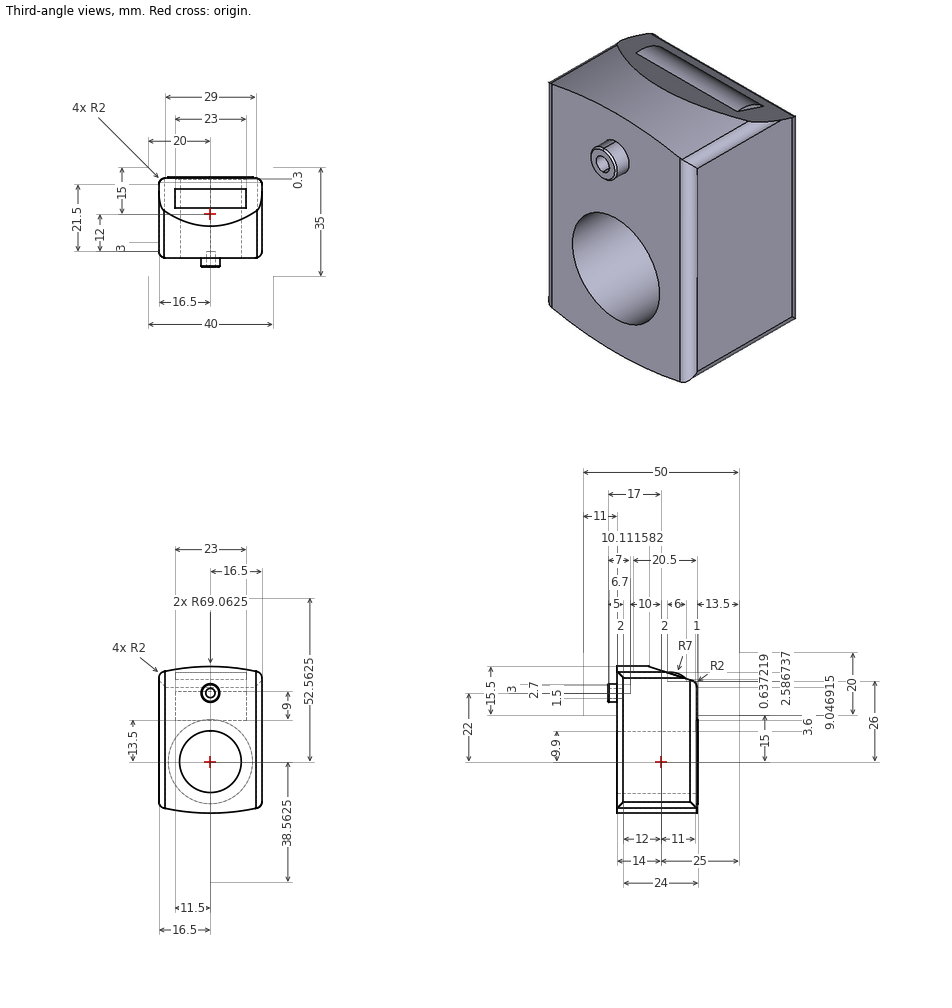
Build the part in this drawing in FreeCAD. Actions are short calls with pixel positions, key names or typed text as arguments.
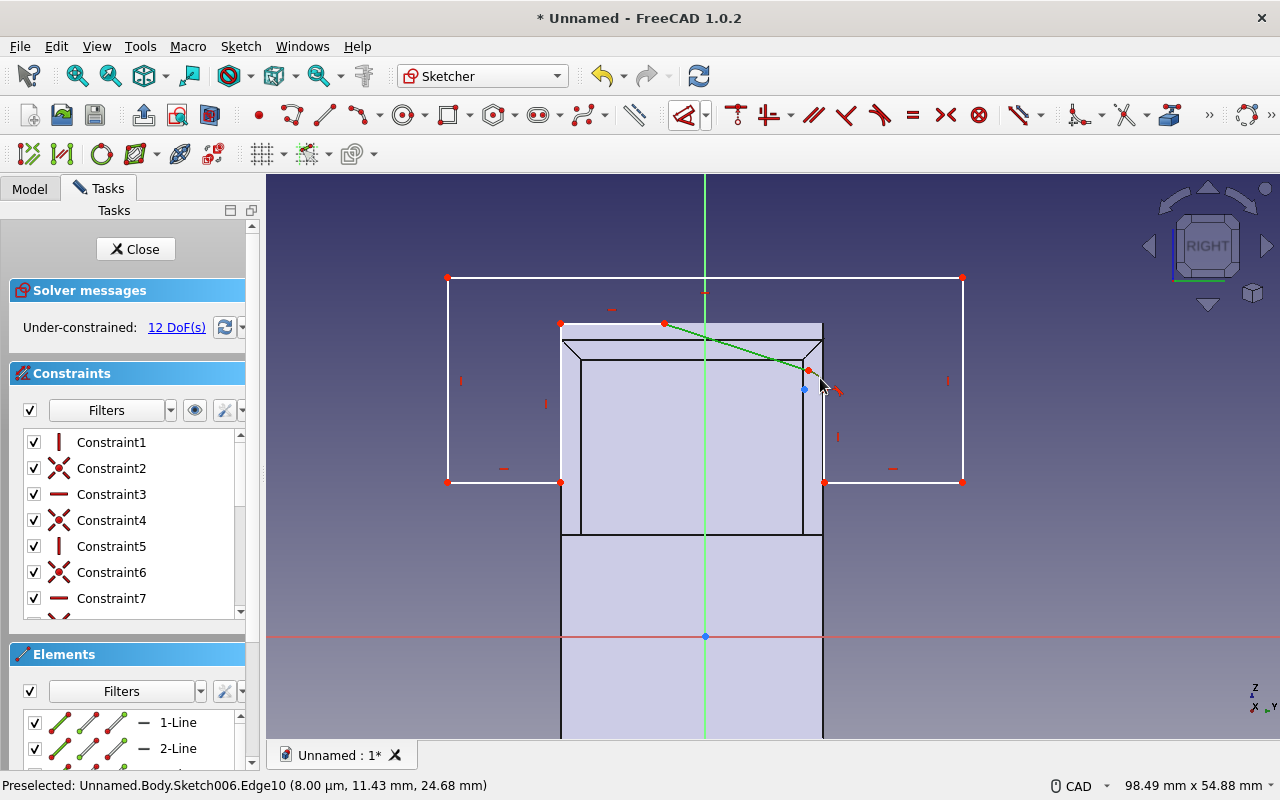
click(880, 116)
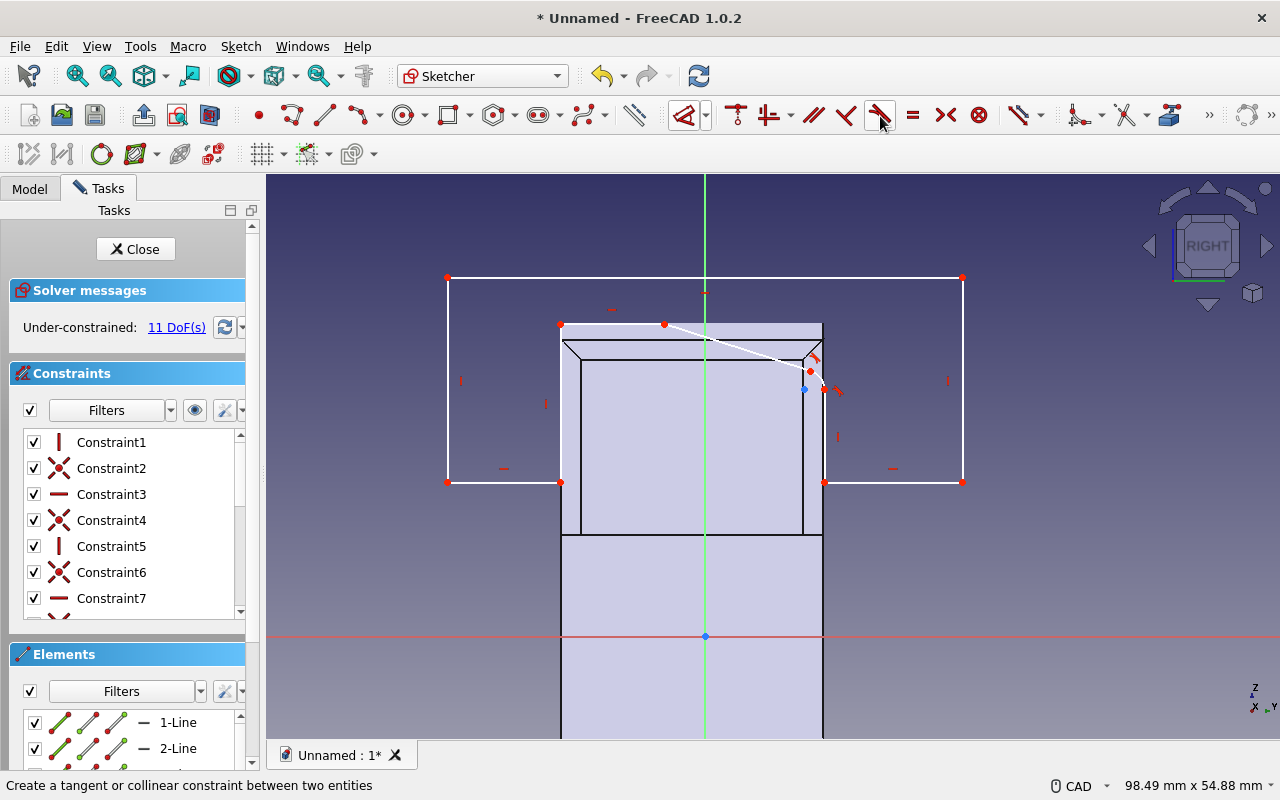
scroll(821, 378, up, 4)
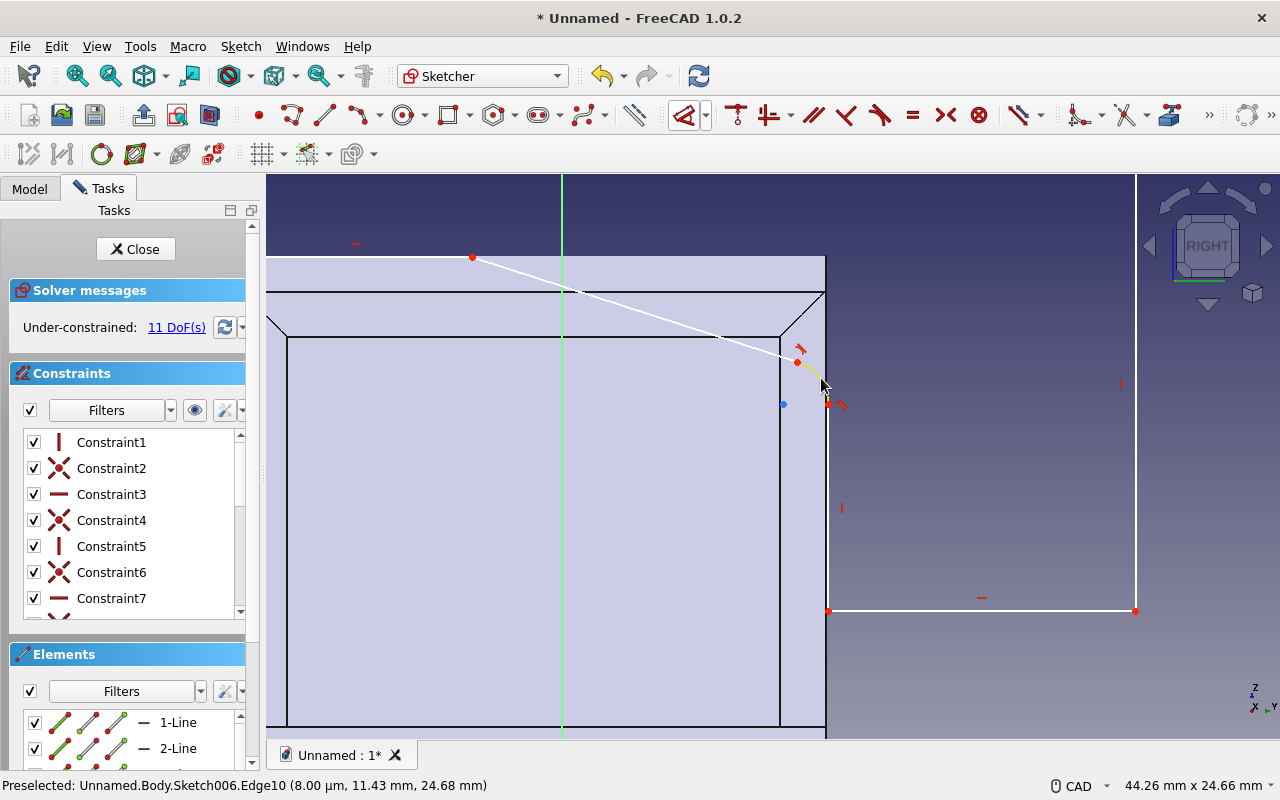
click(820, 378)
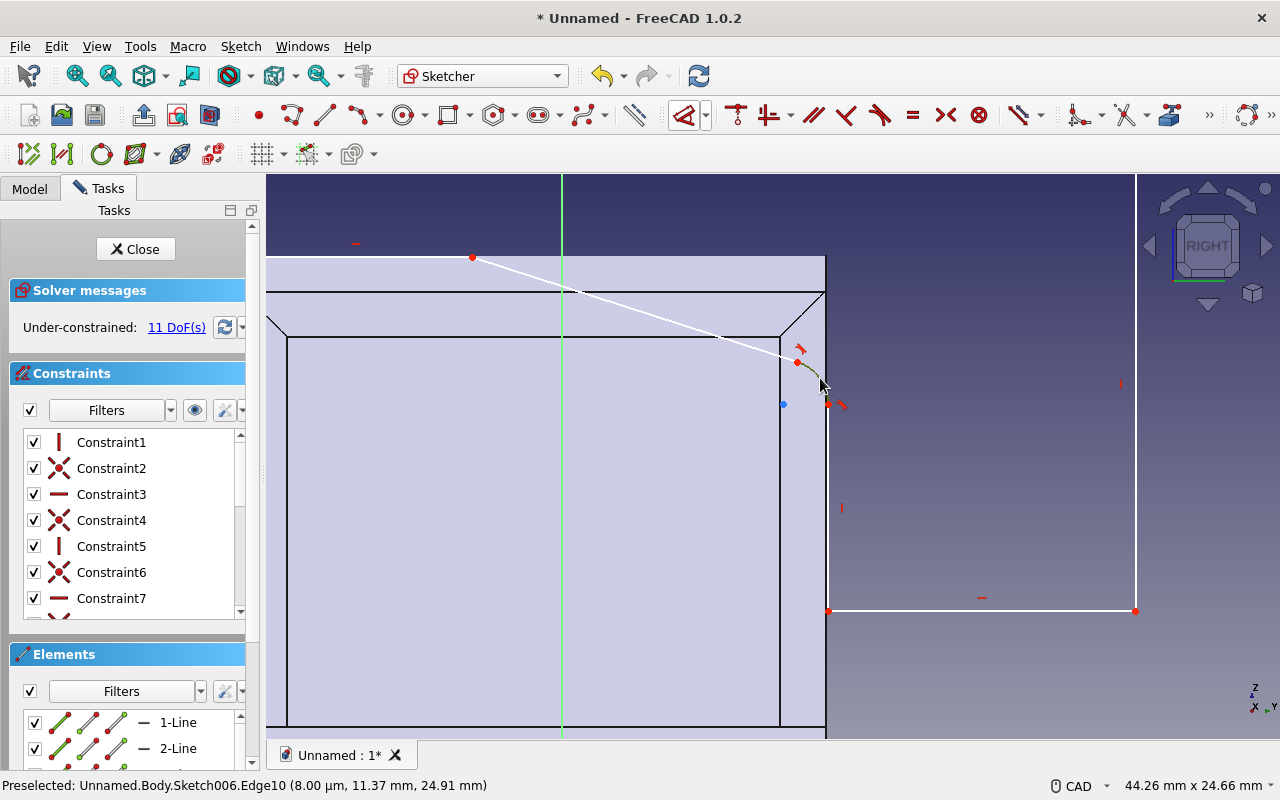
click(706, 116)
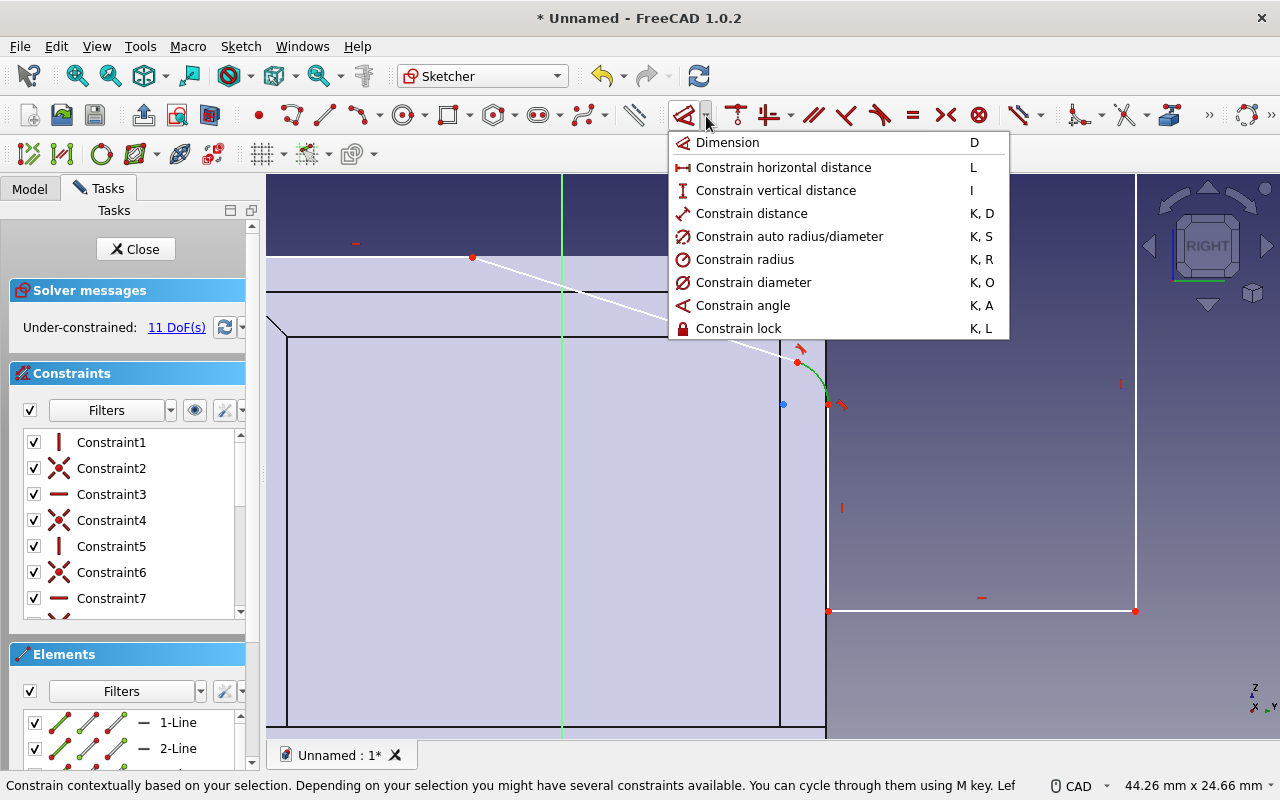
click(839, 260)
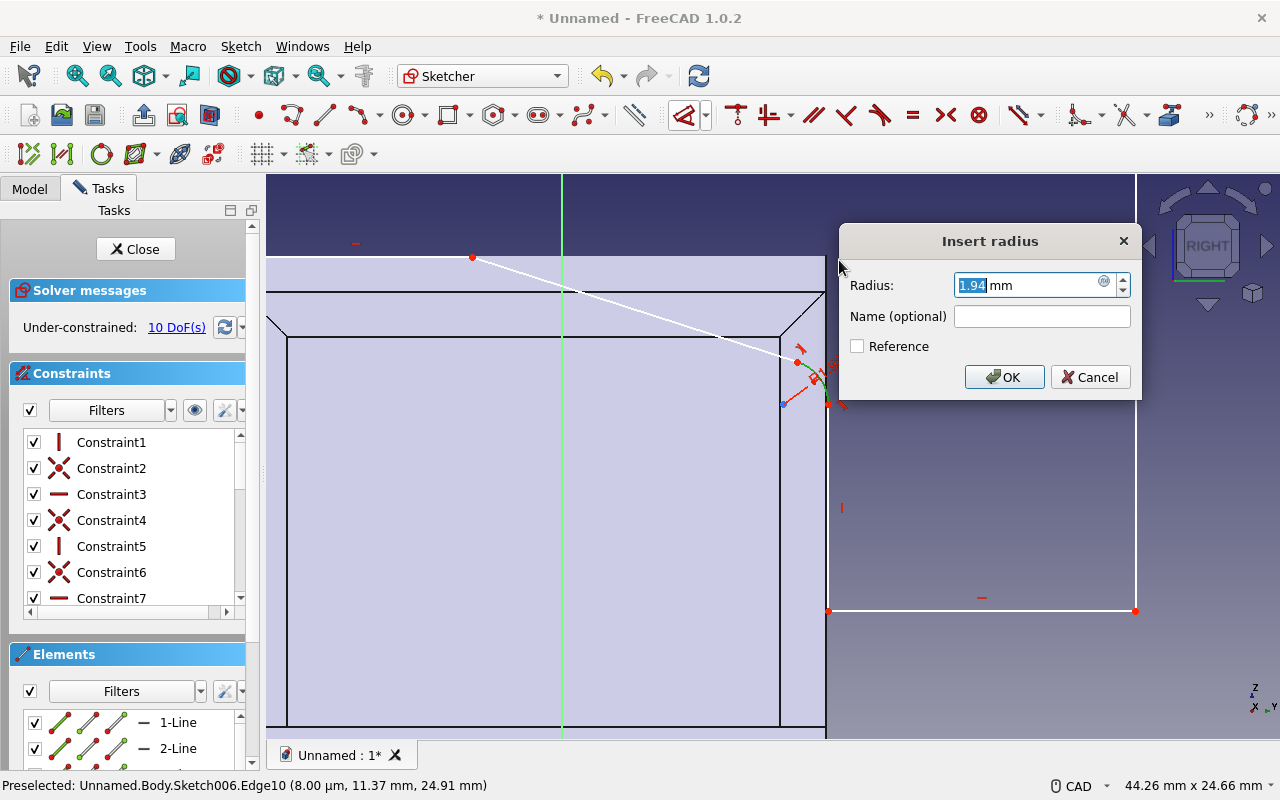
text(2)
key(Return)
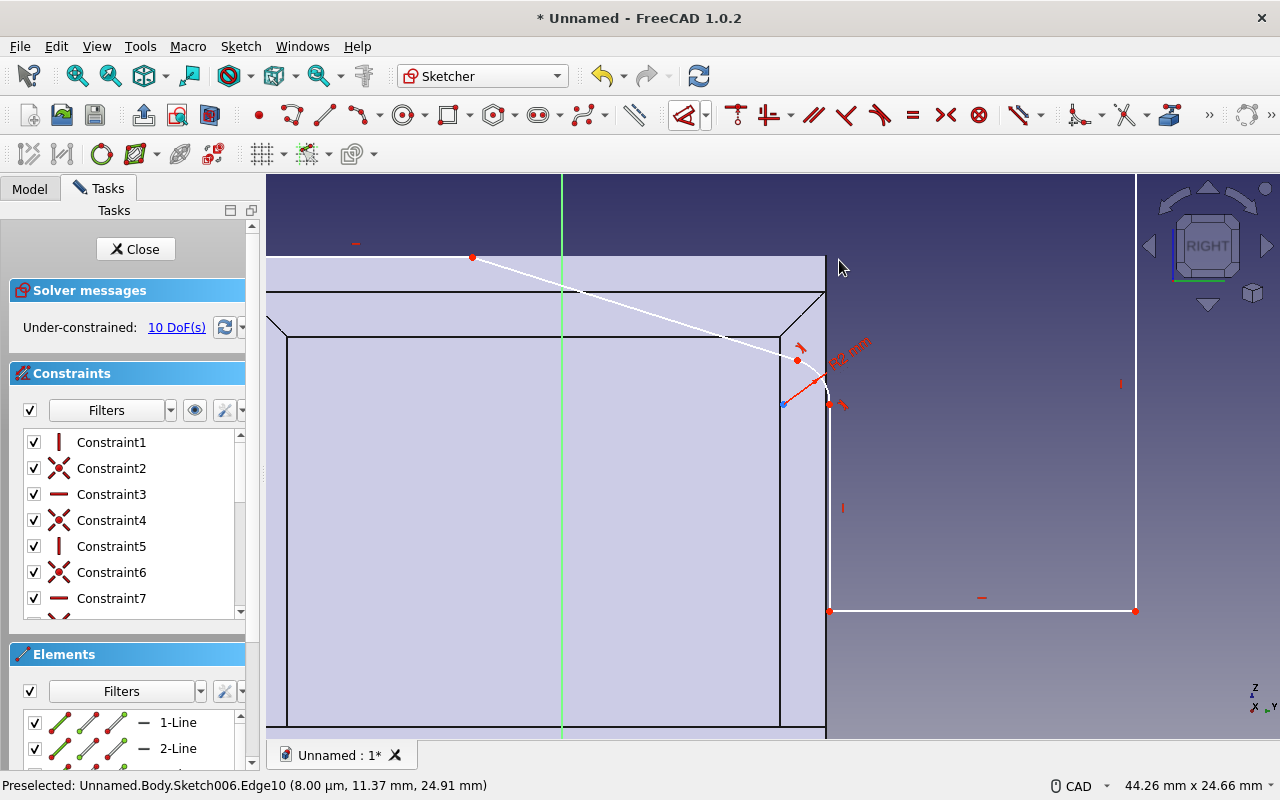
scroll(821, 378, down, 4)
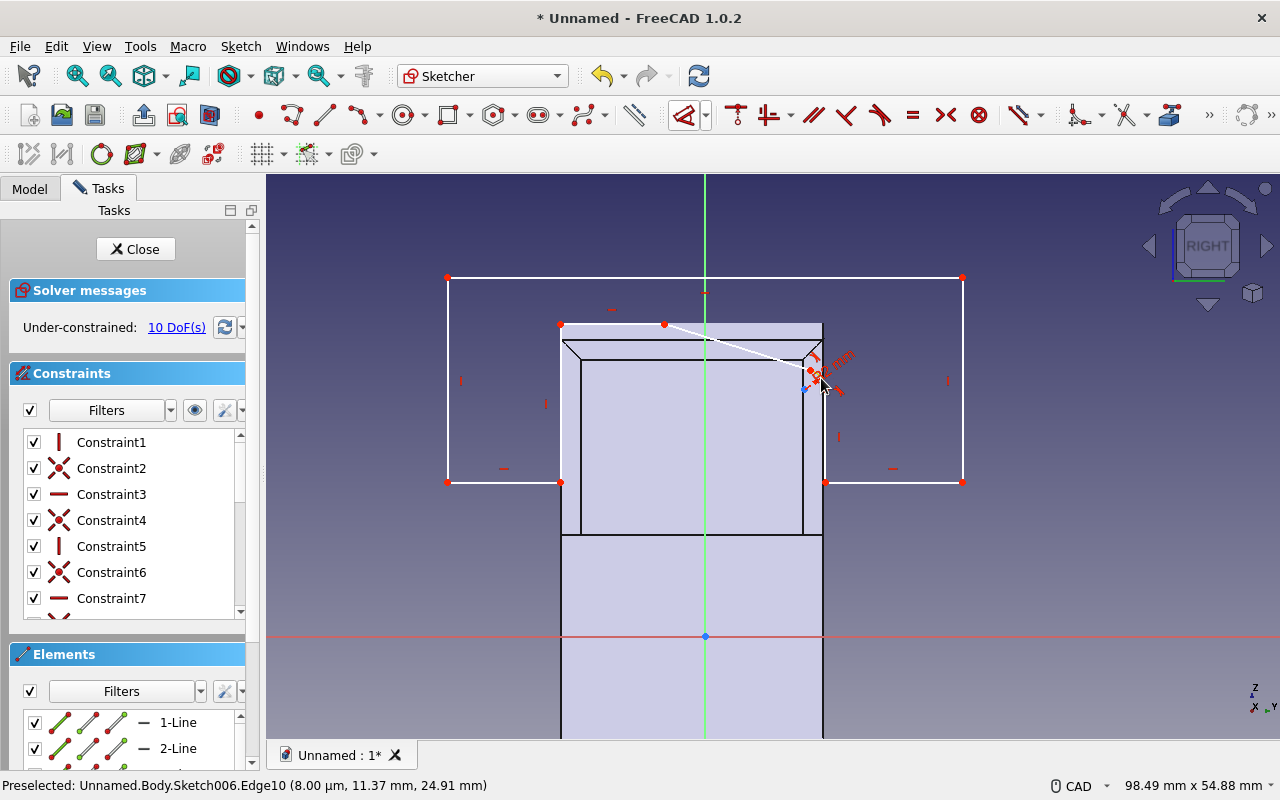
click(963, 422)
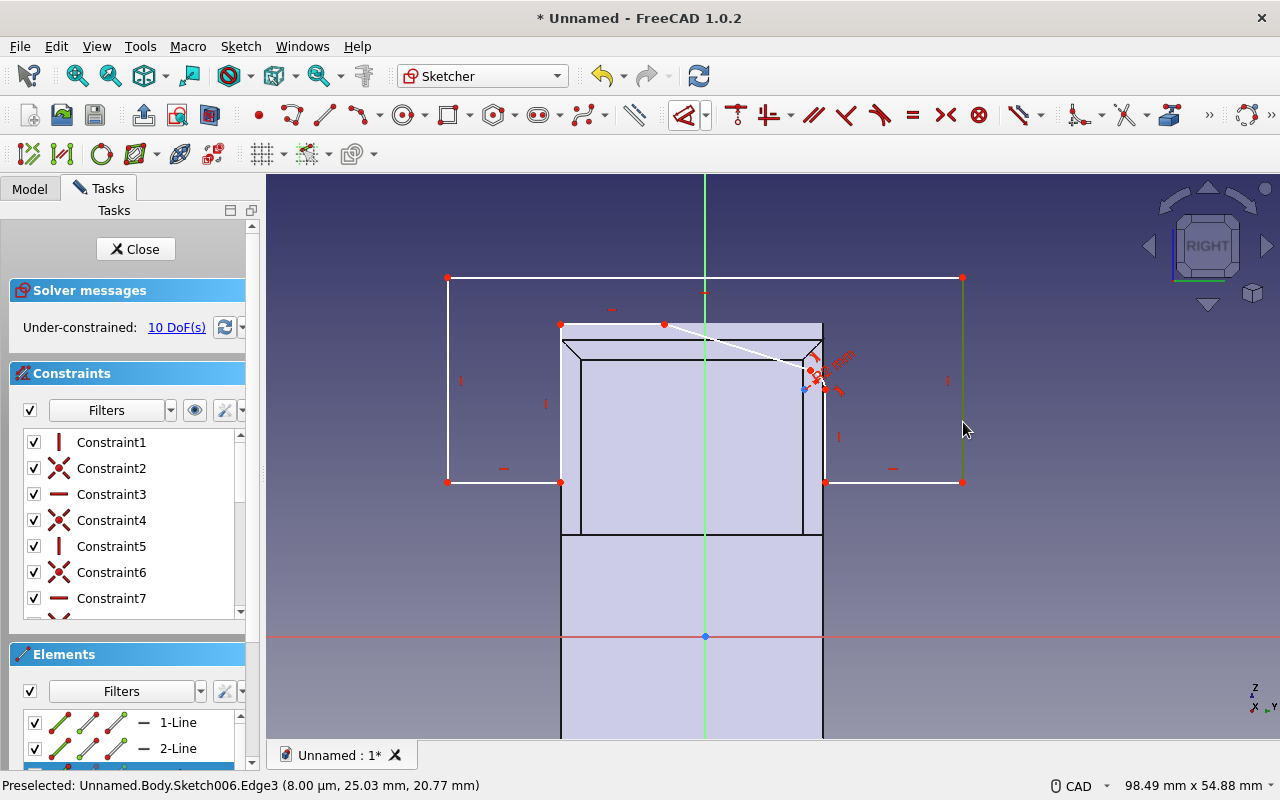
key(i)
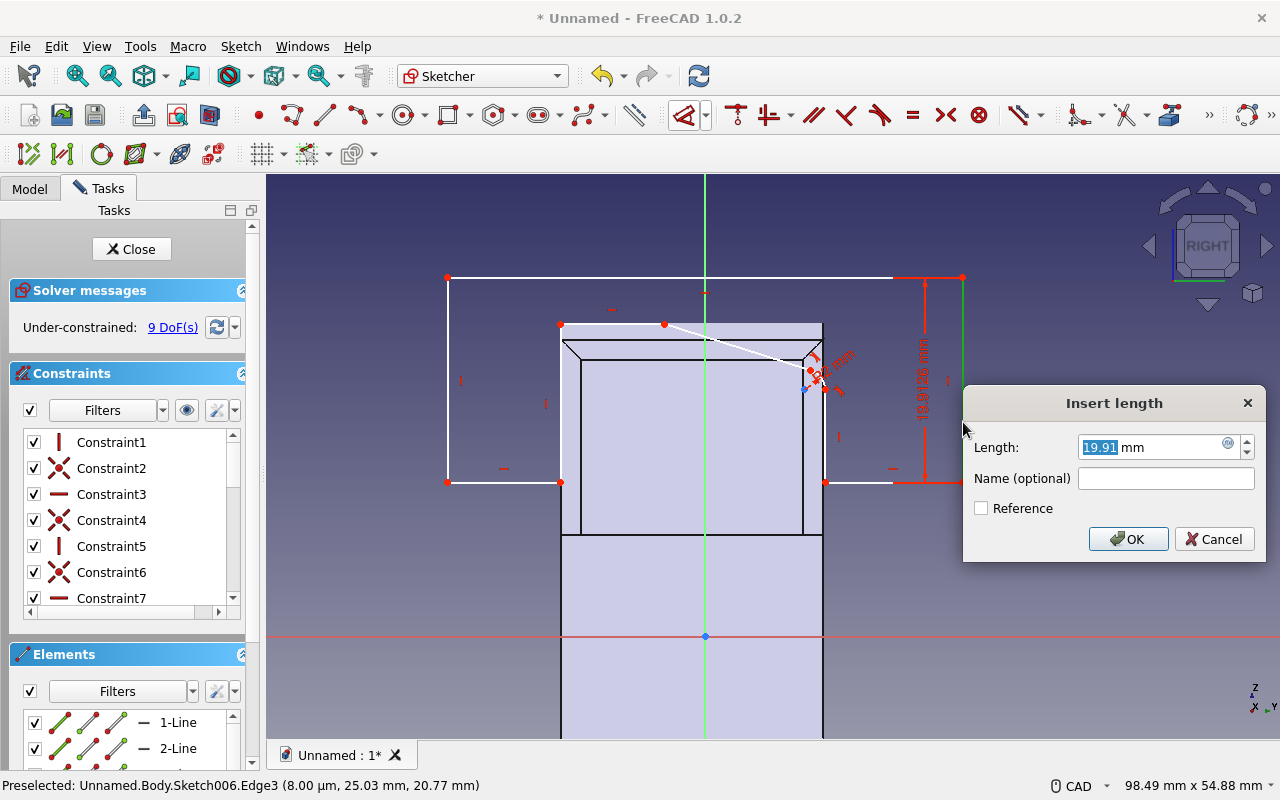
text(20)
key(Return)